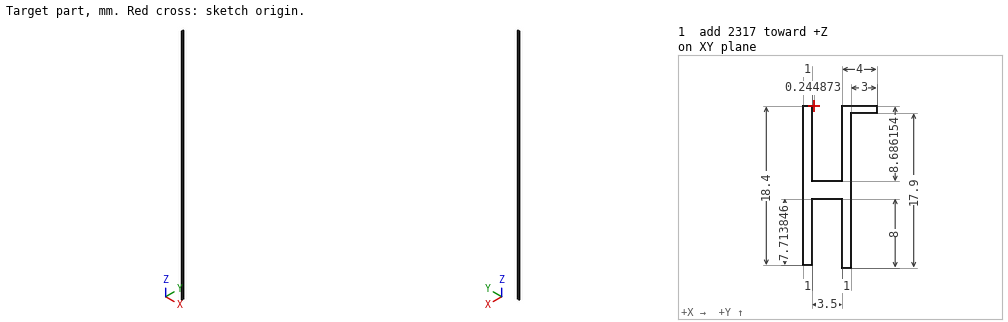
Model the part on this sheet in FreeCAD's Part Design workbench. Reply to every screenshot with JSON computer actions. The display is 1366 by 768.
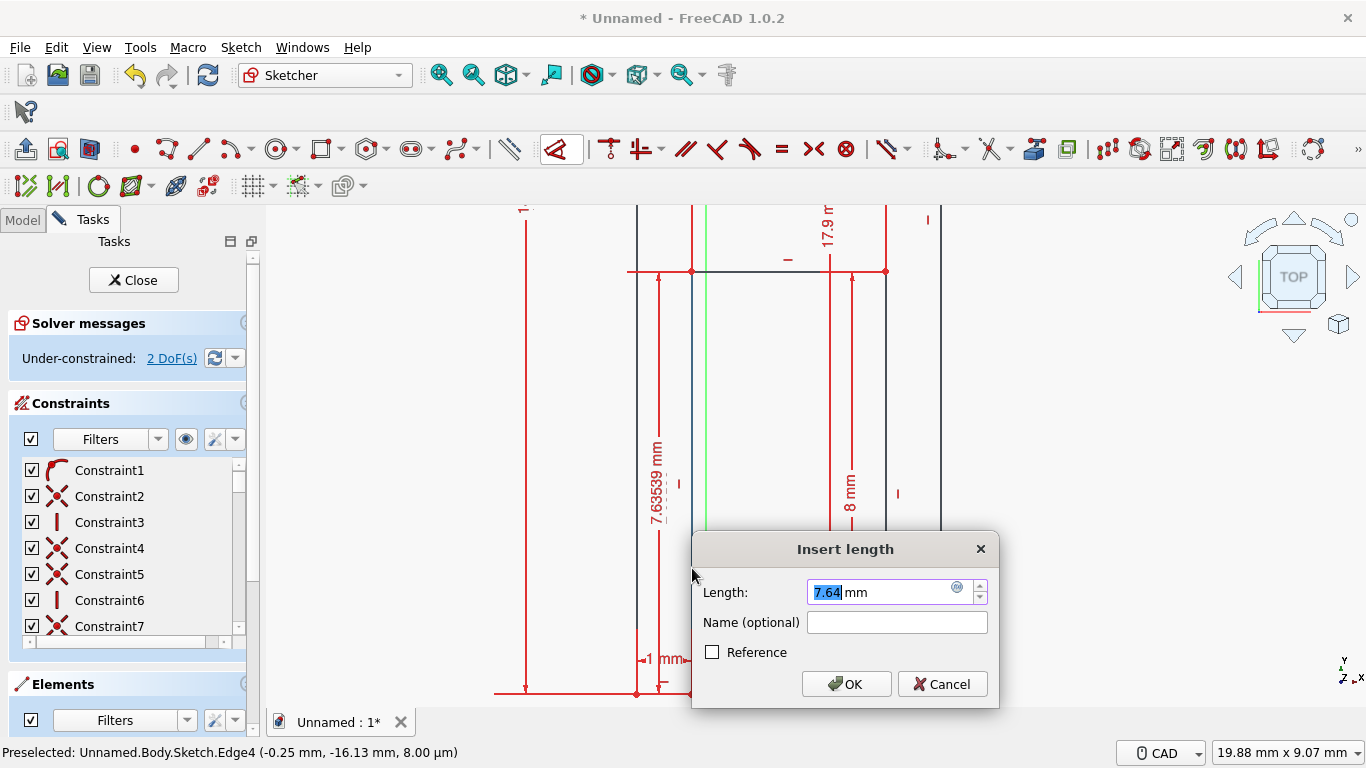
{"action": "type", "text": "7.713846"}
{"action": "key", "text": "Return"}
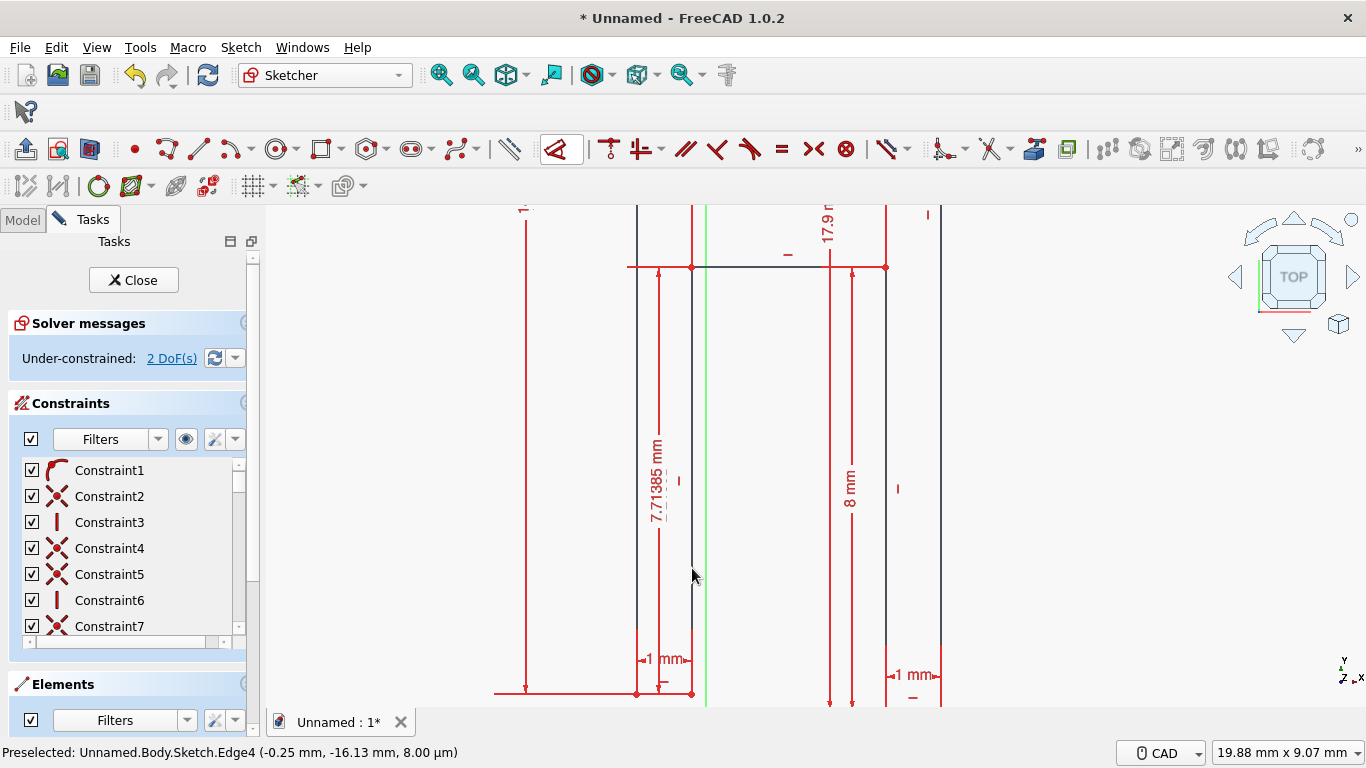
{"action": "scroll", "coordinate": [694, 569], "scroll_direction": "down", "scroll_amount": 6}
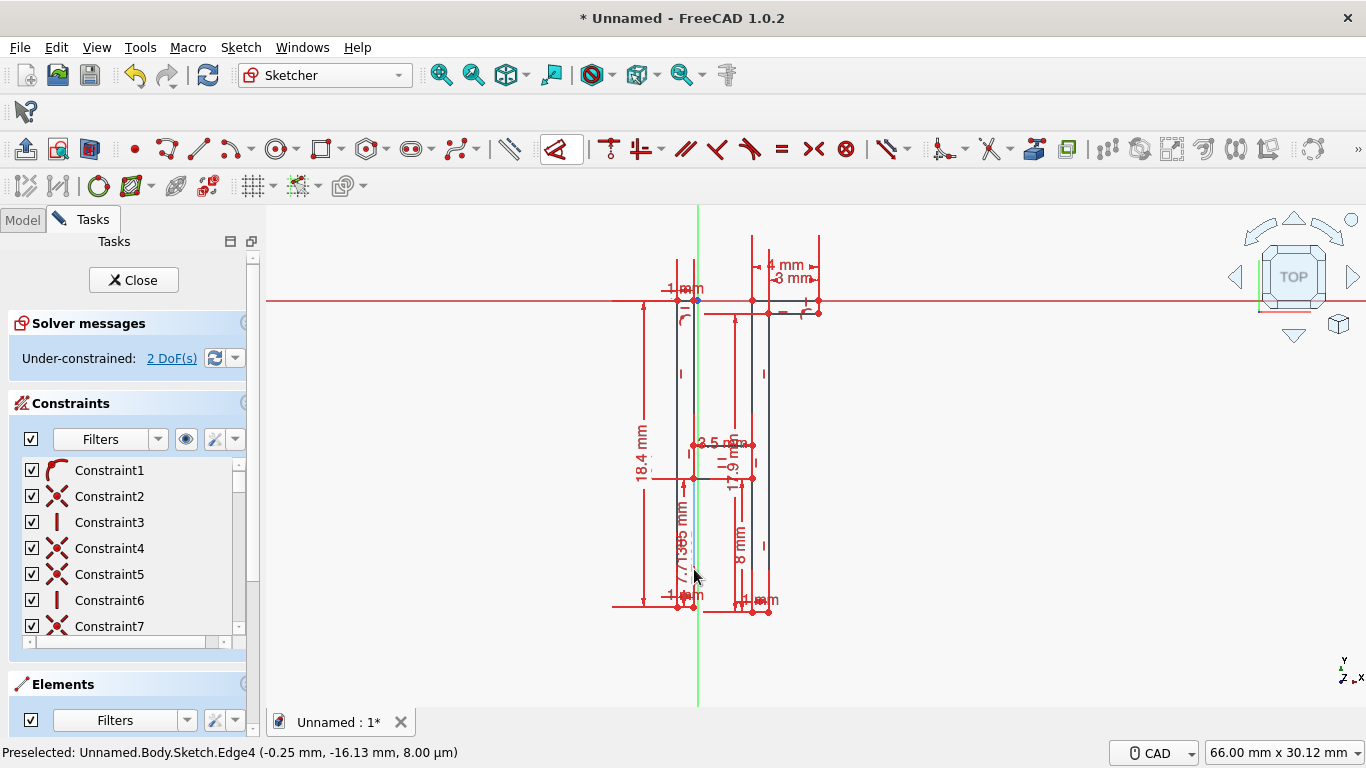
{"action": "left_click", "coordinate": [752, 344]}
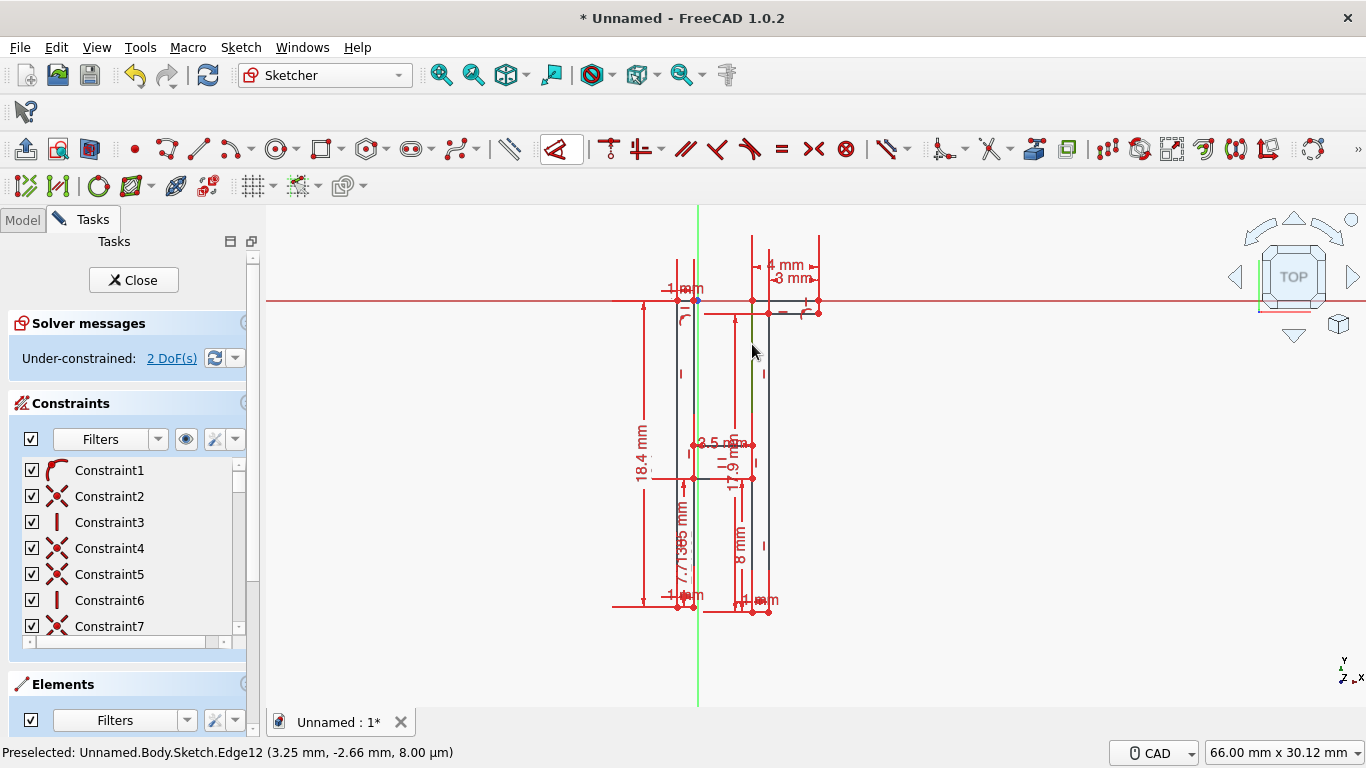
{"action": "key", "text": "i"}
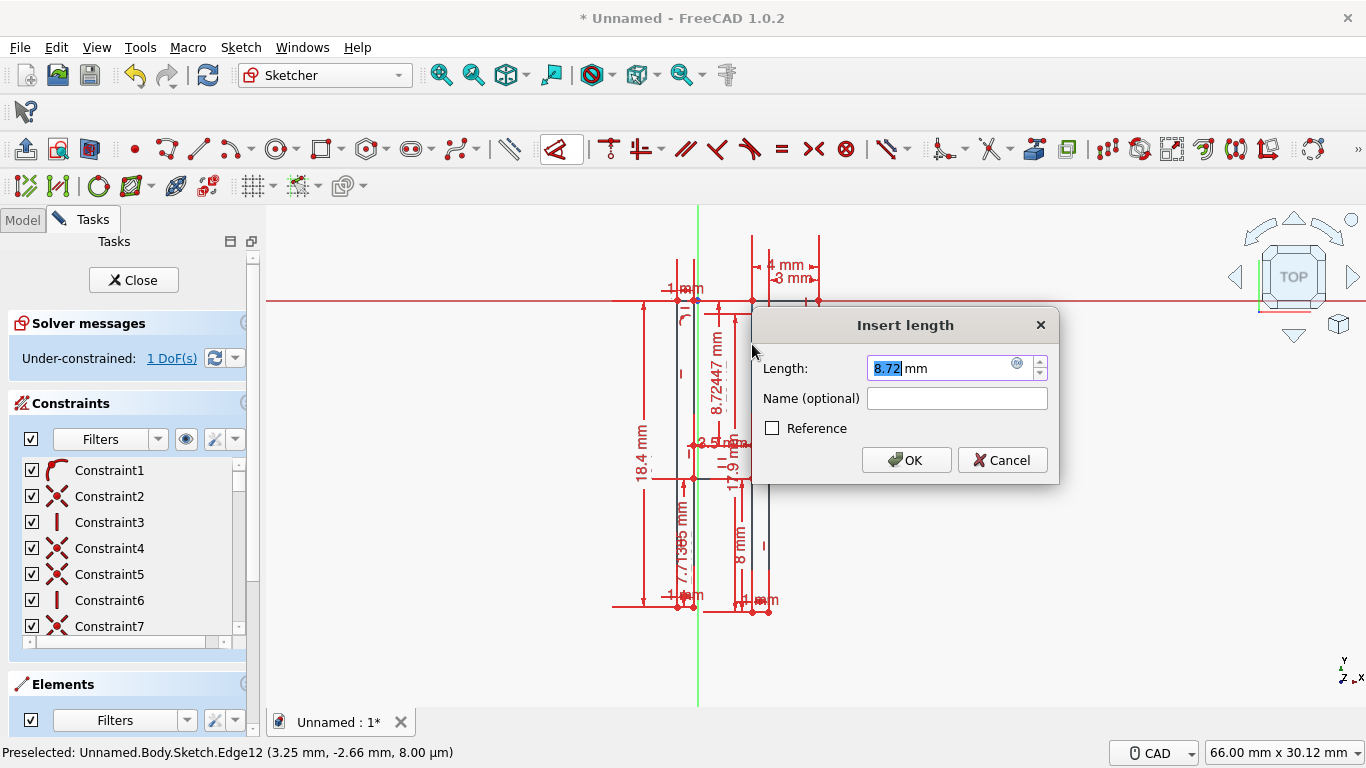
{"action": "type", "text": "8.686154"}
{"action": "key", "text": "Return"}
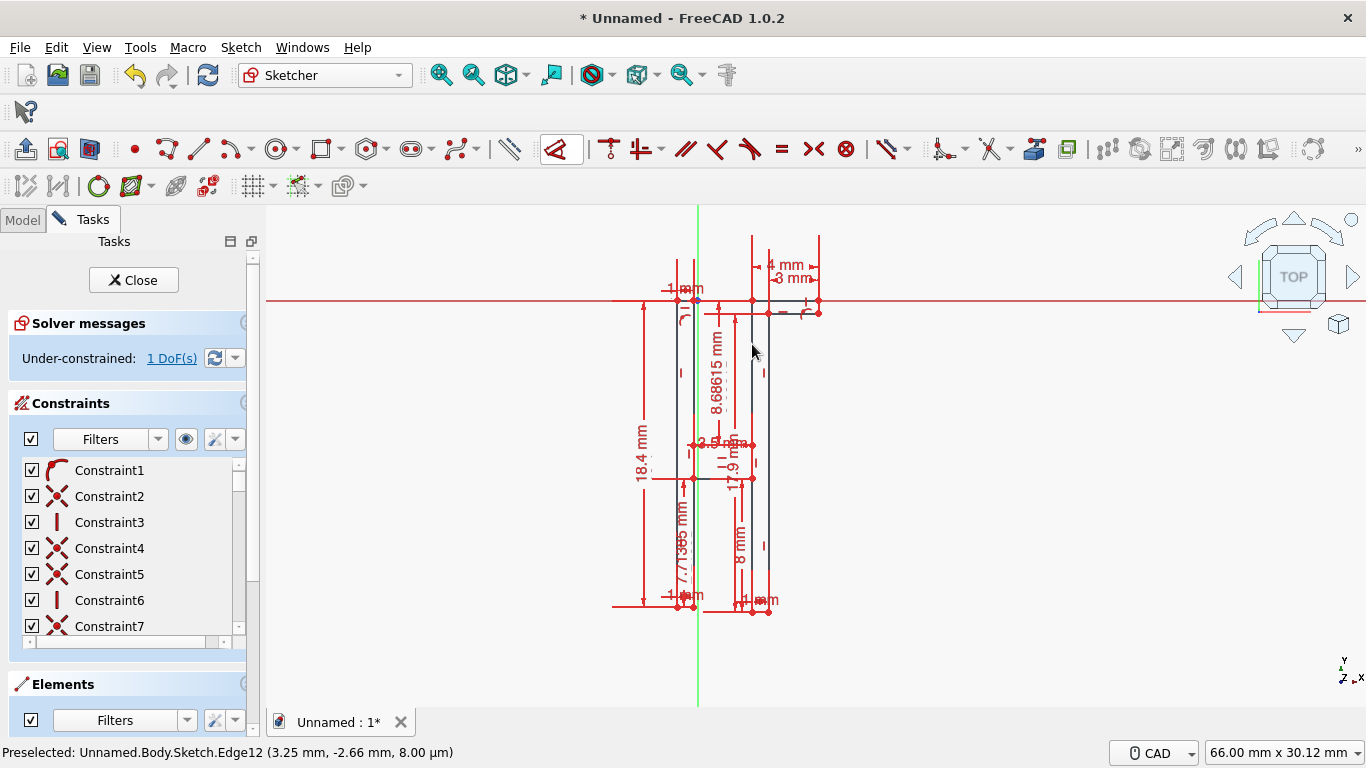
{"action": "scroll", "coordinate": [694, 301], "scroll_direction": "up", "scroll_amount": 12}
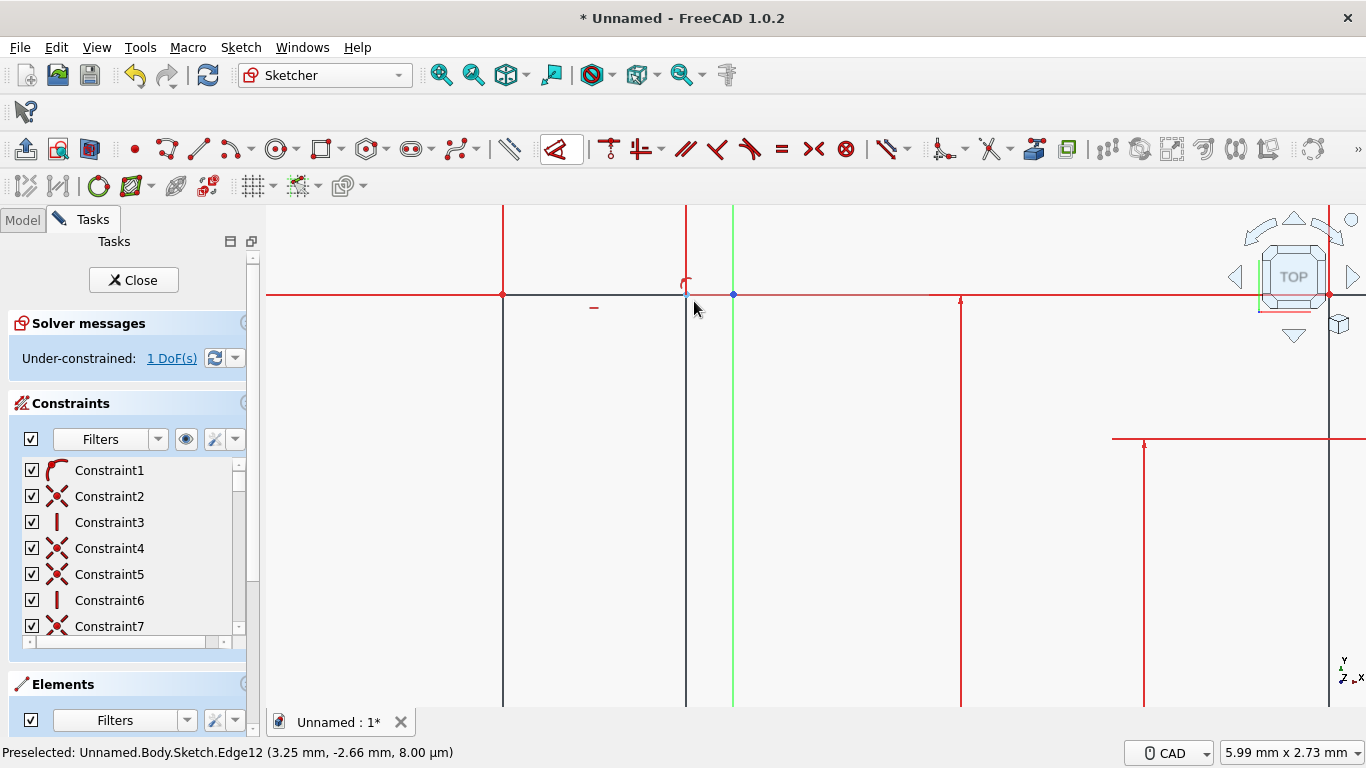
{"action": "left_click", "coordinate": [686, 295]}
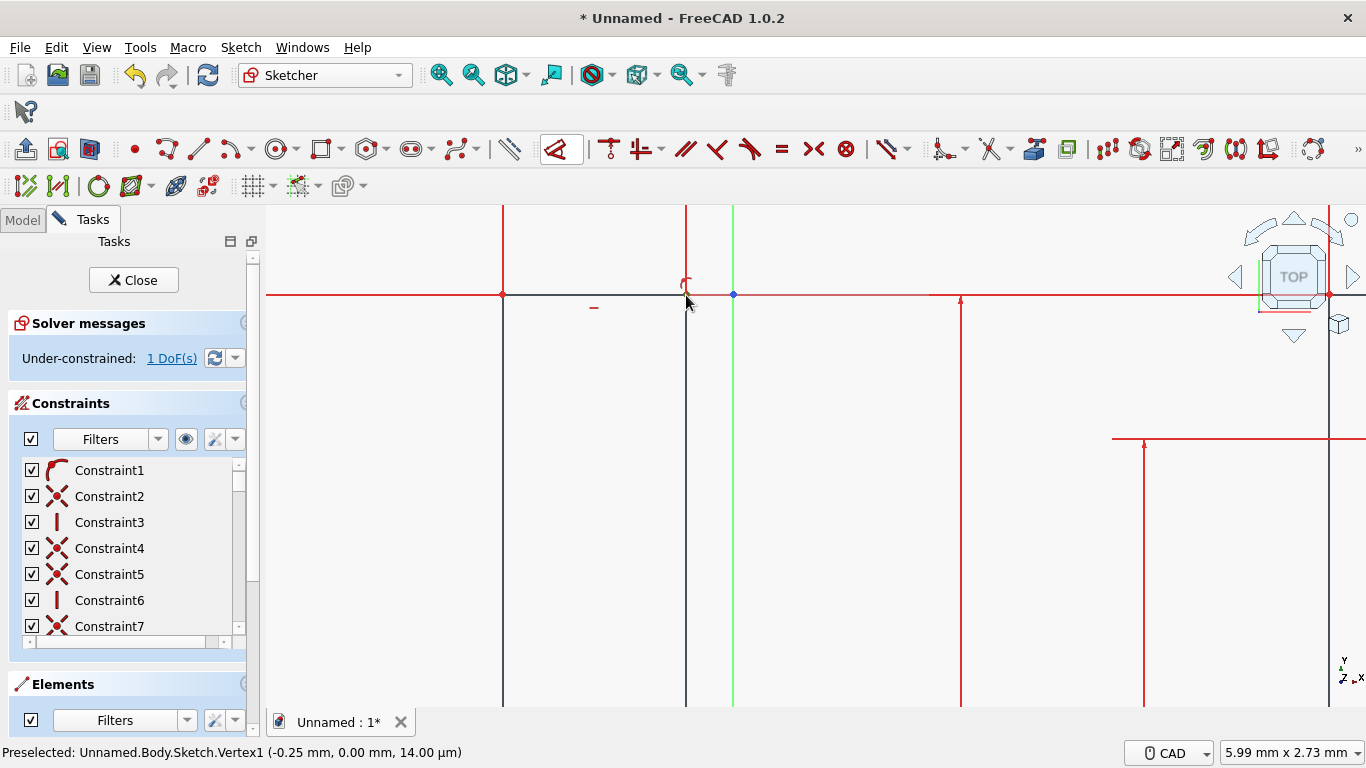
{"action": "key", "text": "l"}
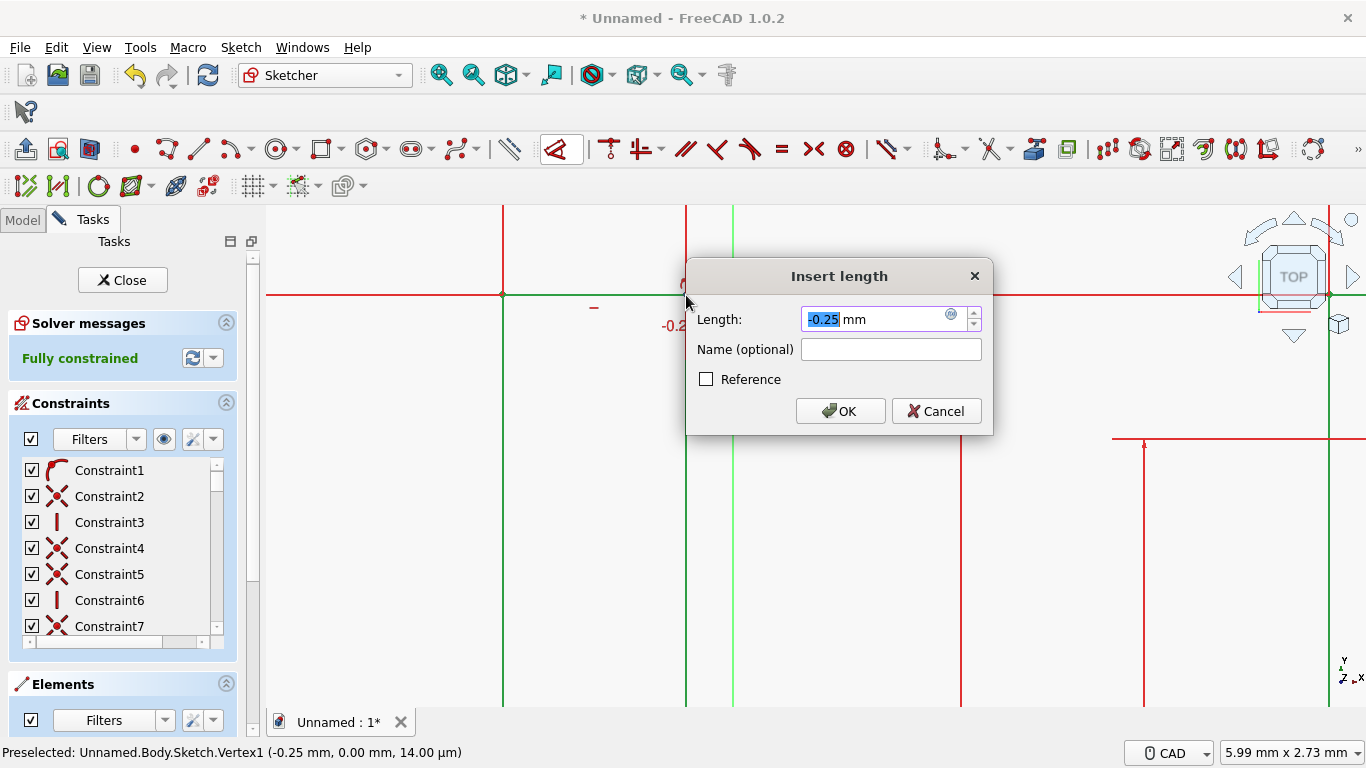
{"action": "type", "text": "-0.244873"}
{"action": "key", "text": "Return"}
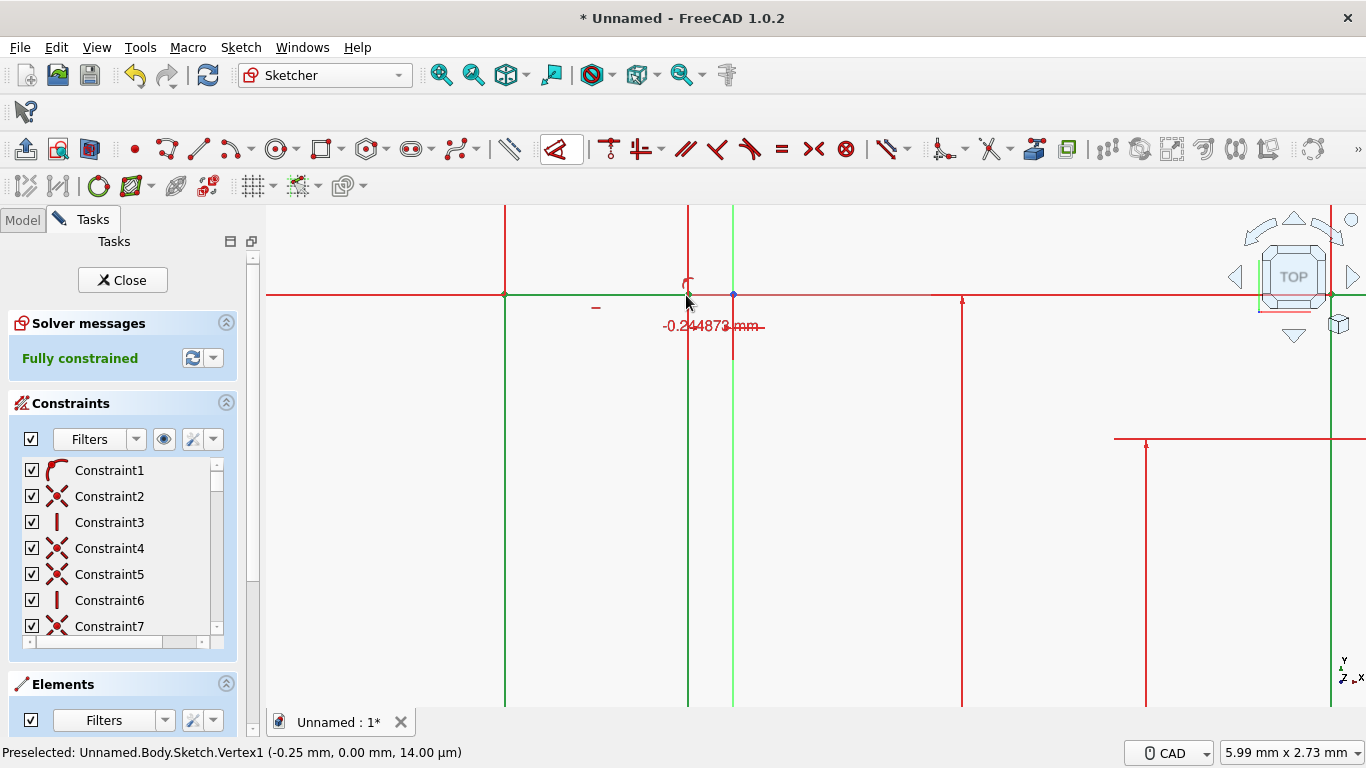
{"action": "left_click", "coordinate": [123, 280]}